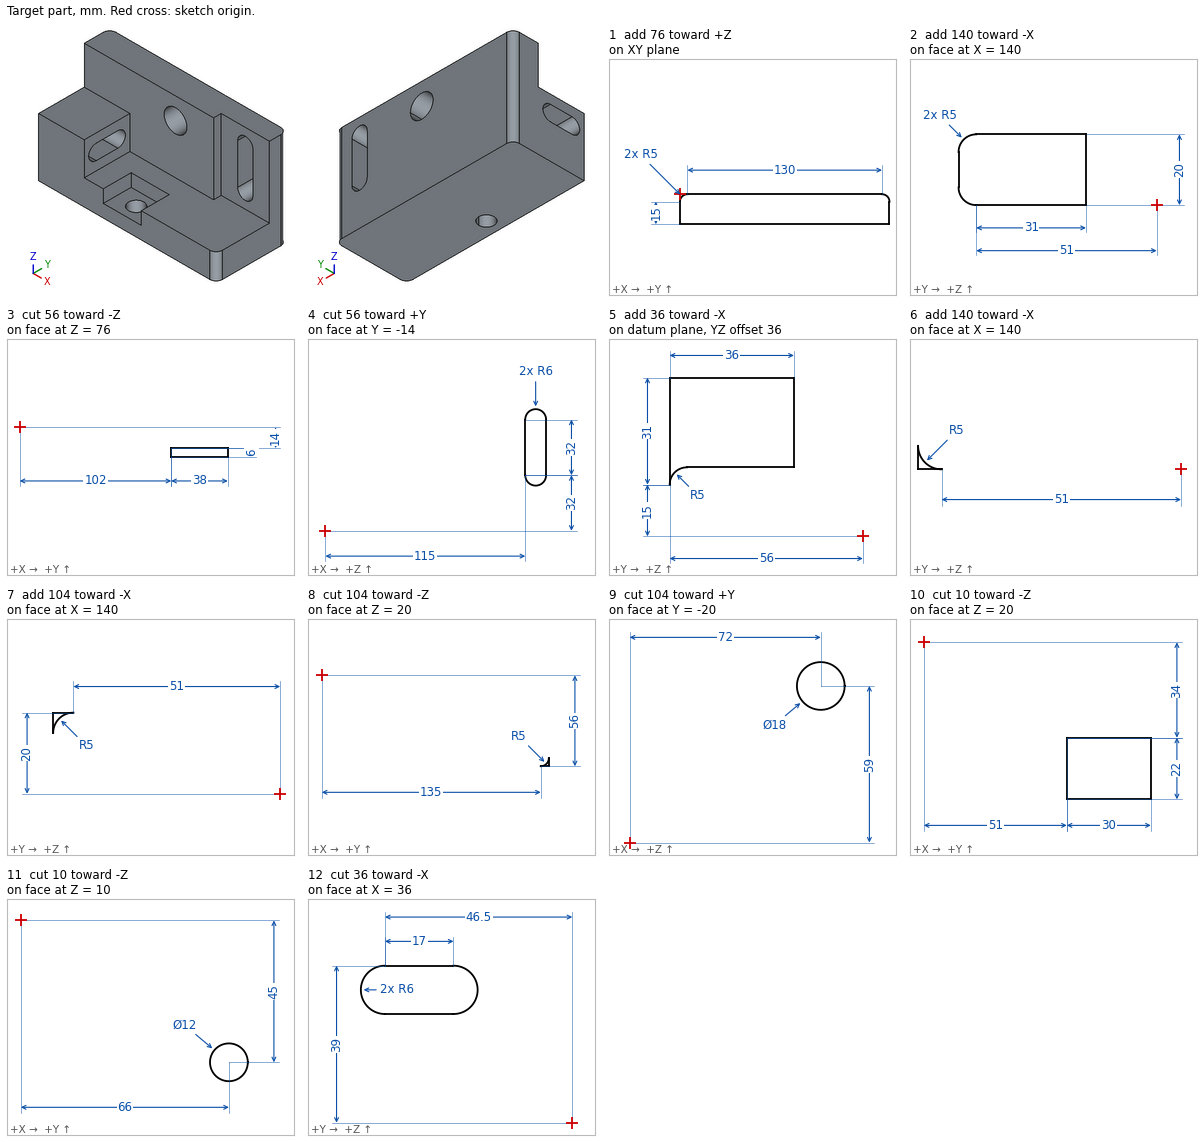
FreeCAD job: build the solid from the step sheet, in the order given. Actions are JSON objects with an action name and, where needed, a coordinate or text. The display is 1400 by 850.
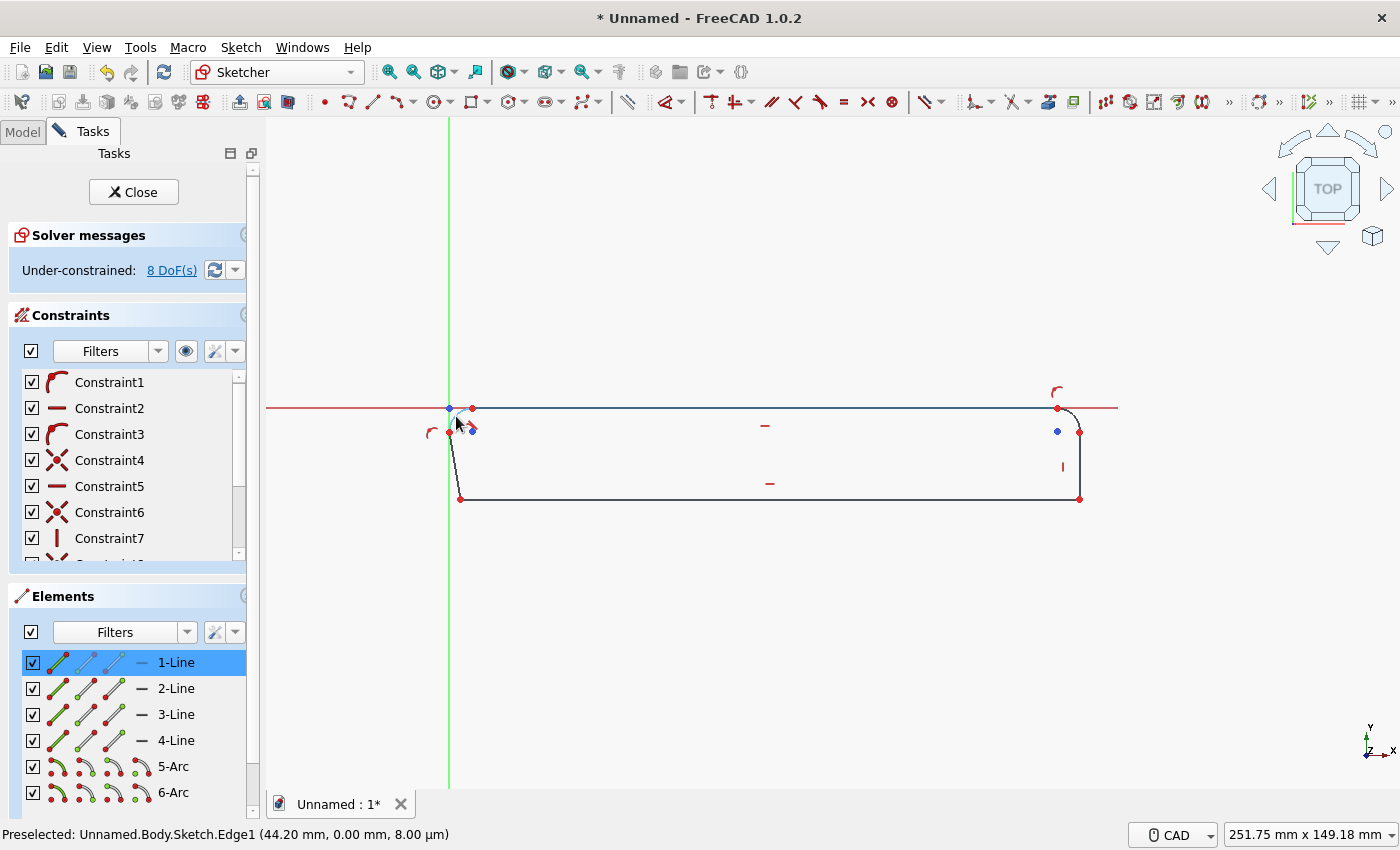
{"action": "scroll", "coordinate": [1078, 422], "scroll_direction": "up", "scroll_amount": 2}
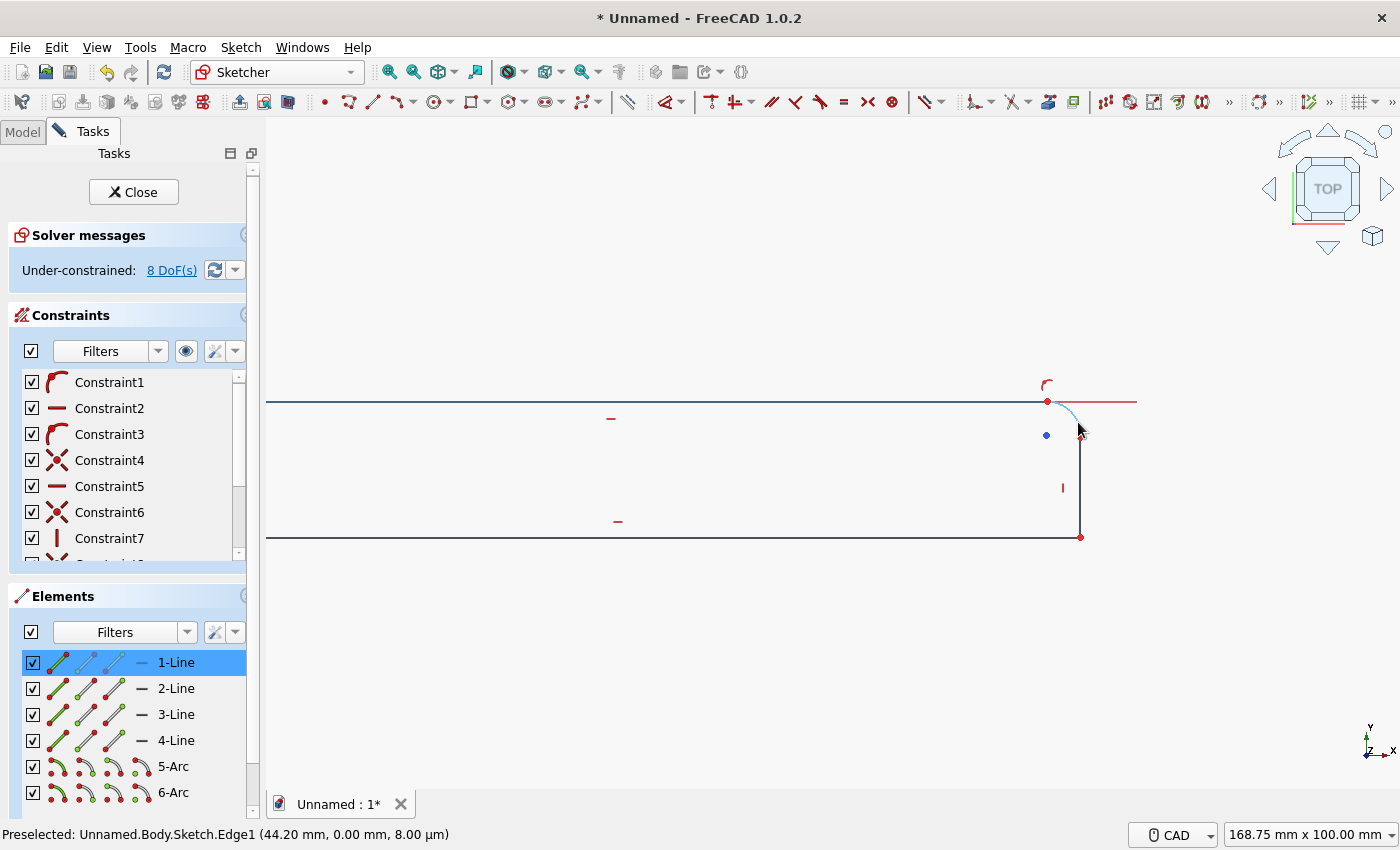
{"action": "left_click", "coordinate": [1078, 422]}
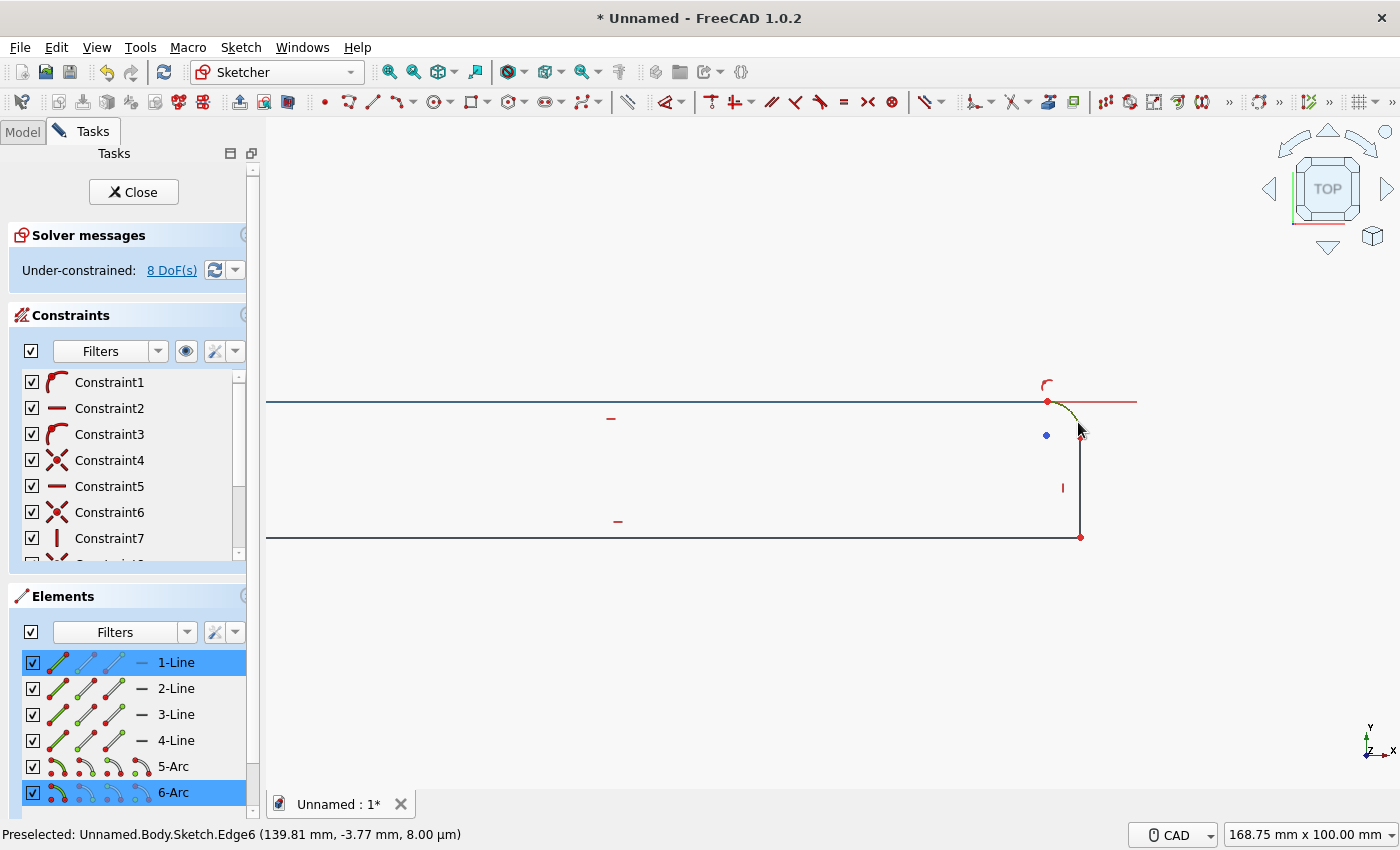
{"action": "left_click", "coordinate": [820, 102]}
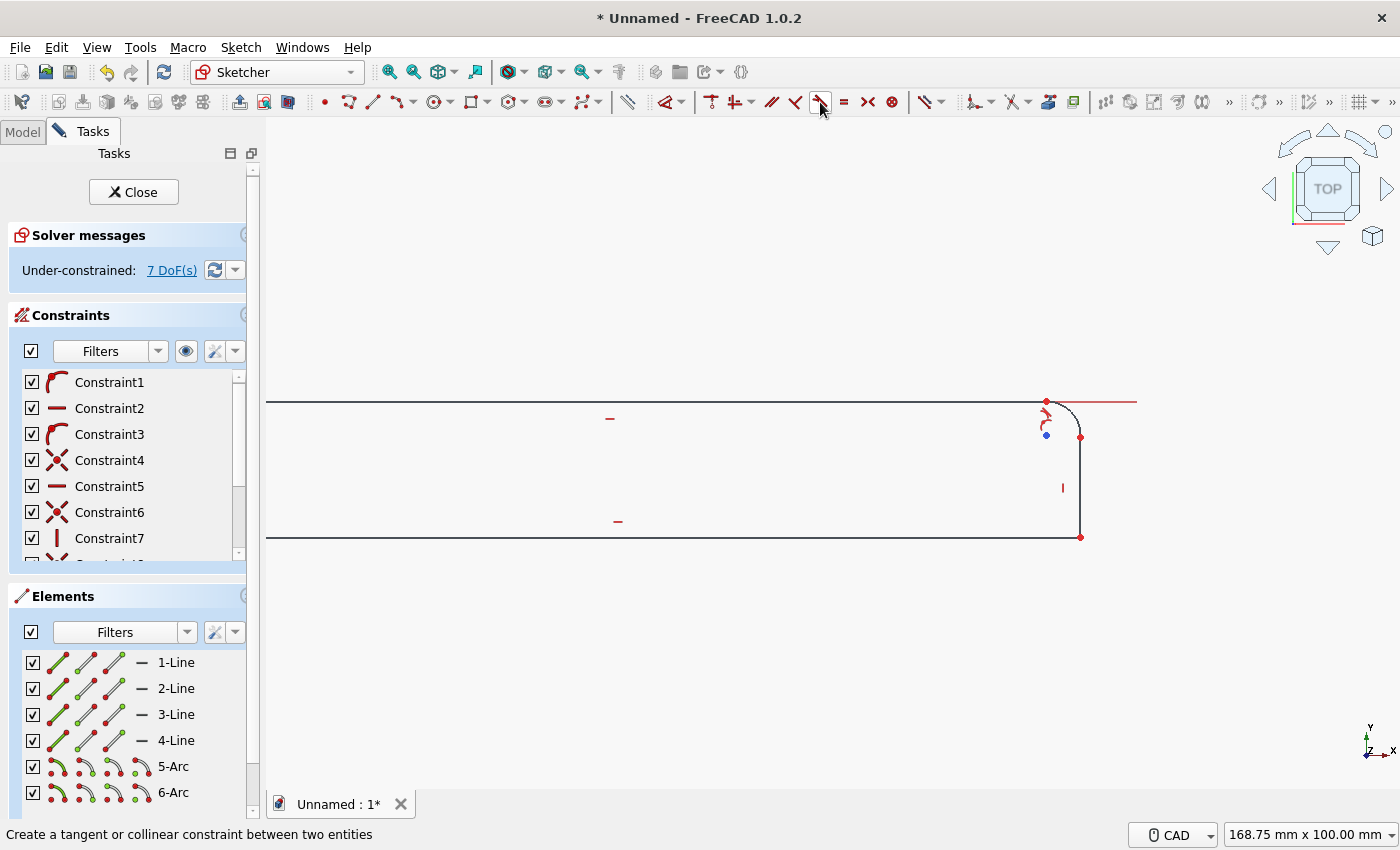
{"action": "scroll", "coordinate": [1078, 421], "scroll_direction": "down", "scroll_amount": 2}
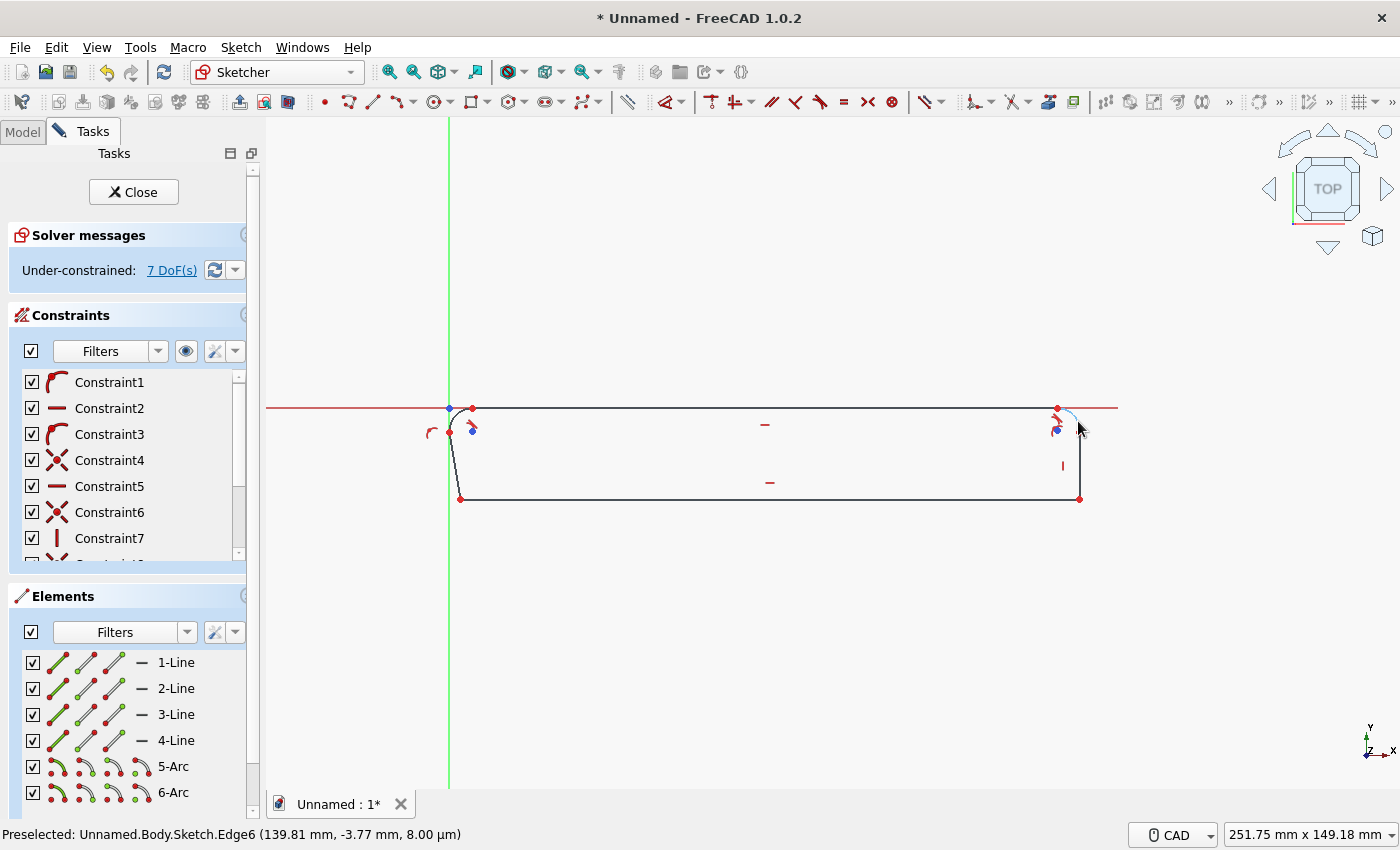
{"action": "scroll", "coordinate": [457, 479], "scroll_direction": "up", "scroll_amount": 3}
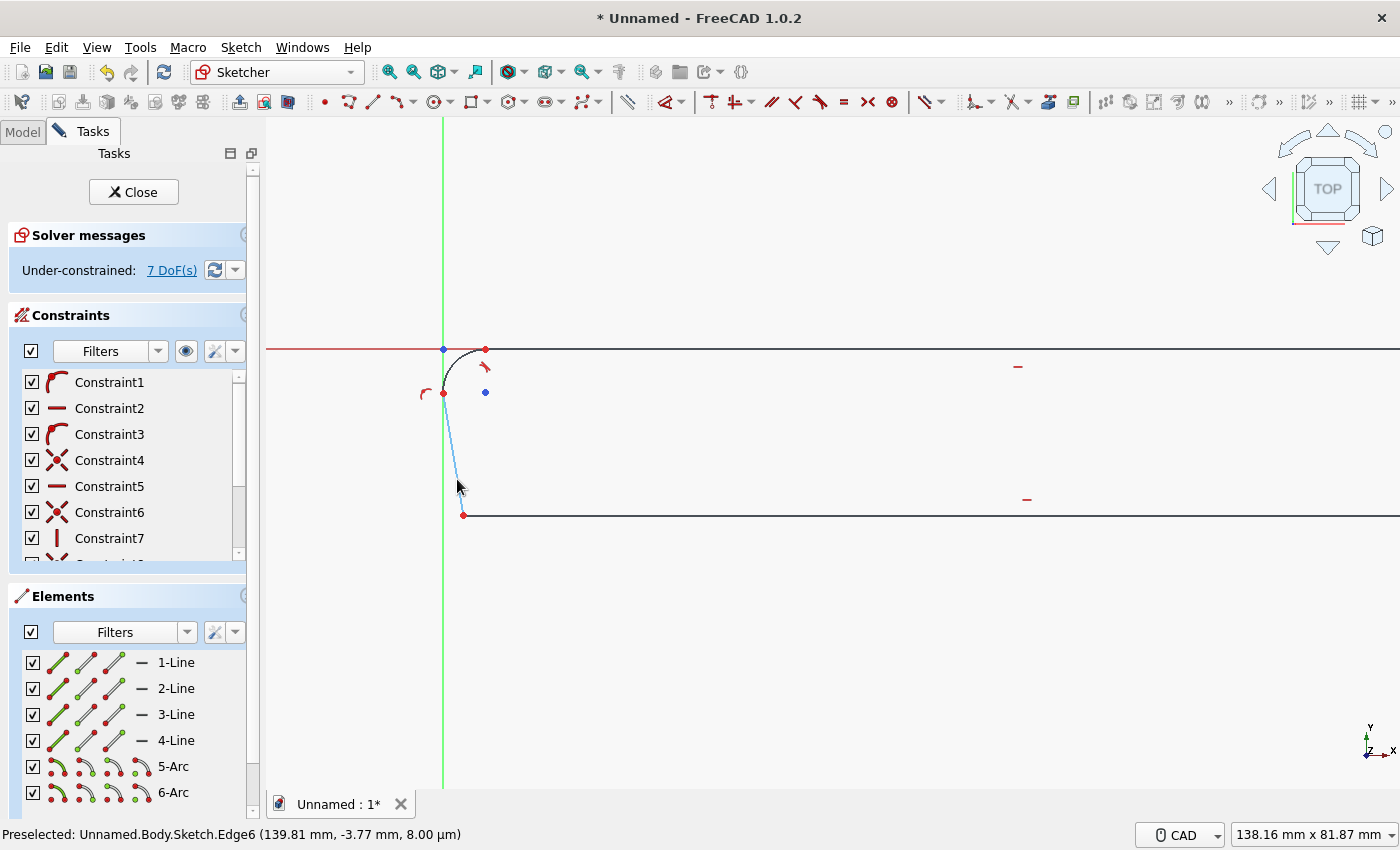
{"action": "left_click", "coordinate": [457, 479]}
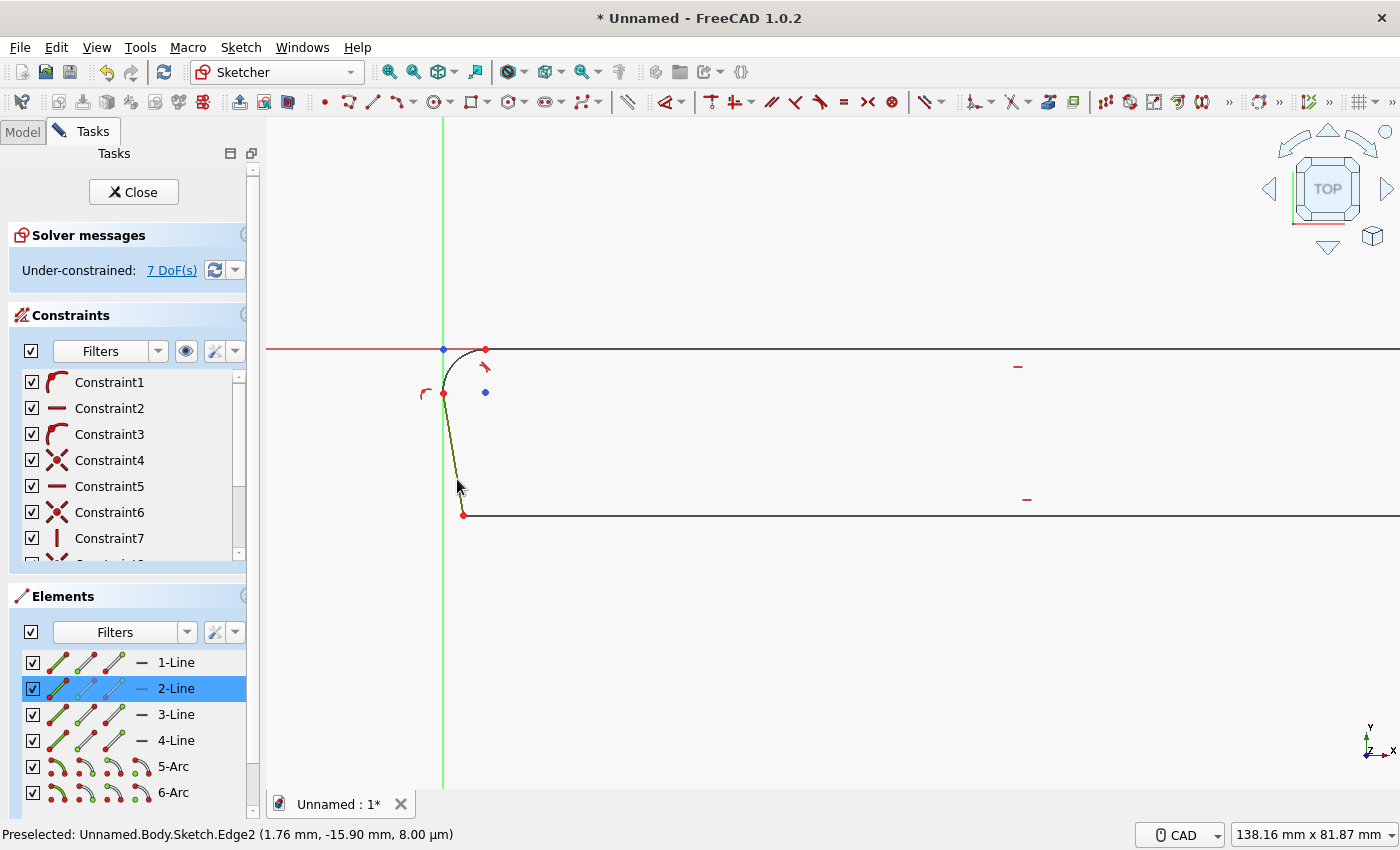
{"action": "left_click", "coordinate": [455, 362]}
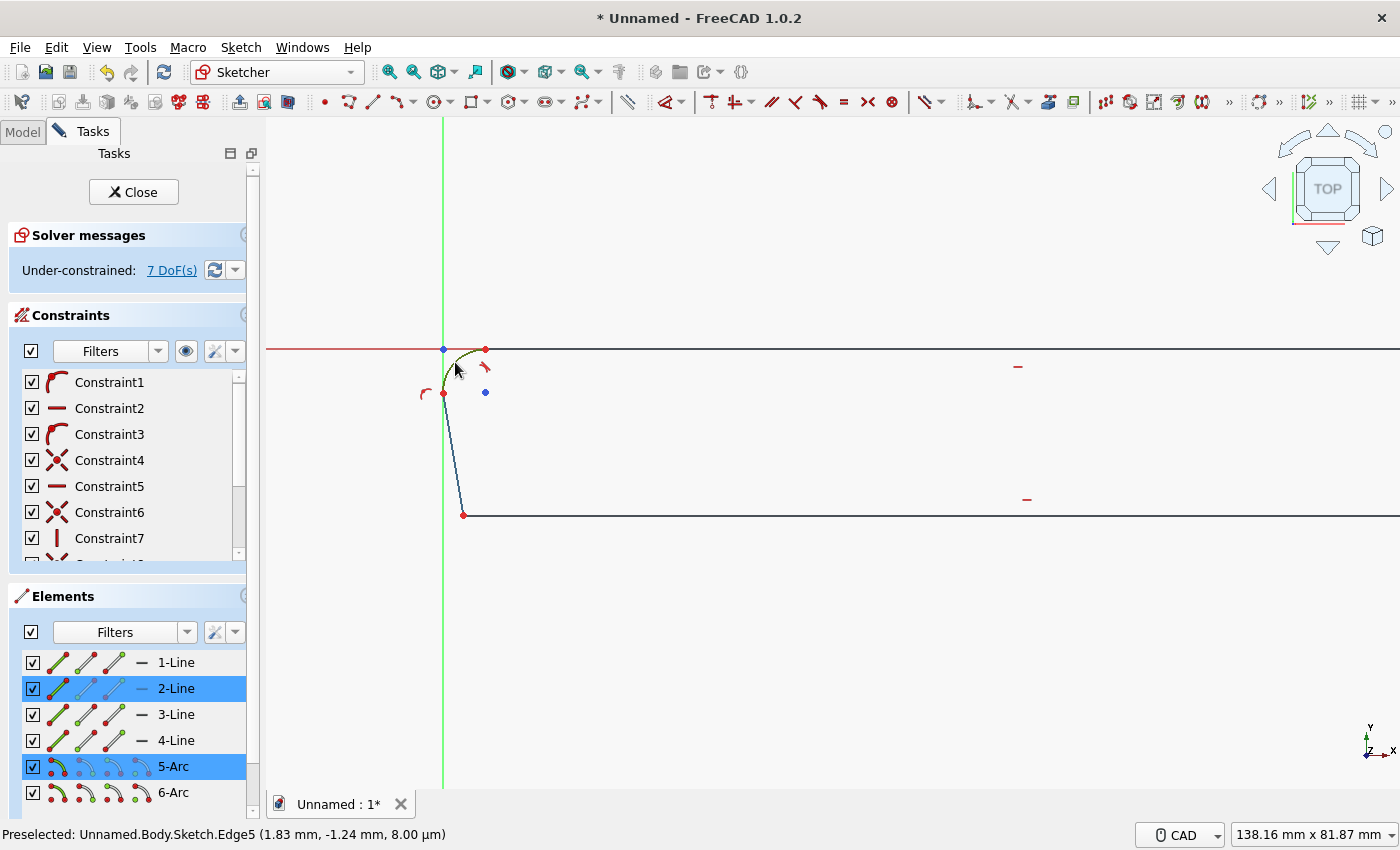
{"action": "left_click", "coordinate": [820, 102]}